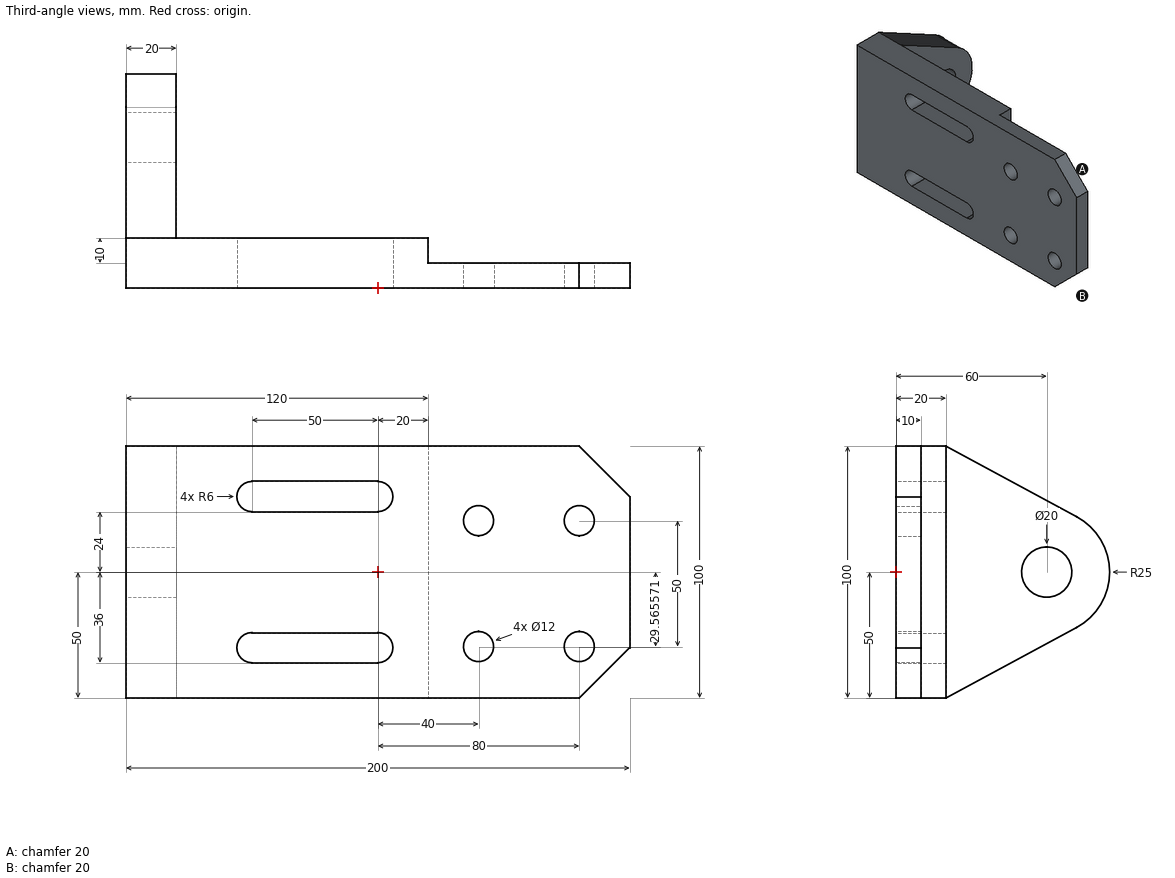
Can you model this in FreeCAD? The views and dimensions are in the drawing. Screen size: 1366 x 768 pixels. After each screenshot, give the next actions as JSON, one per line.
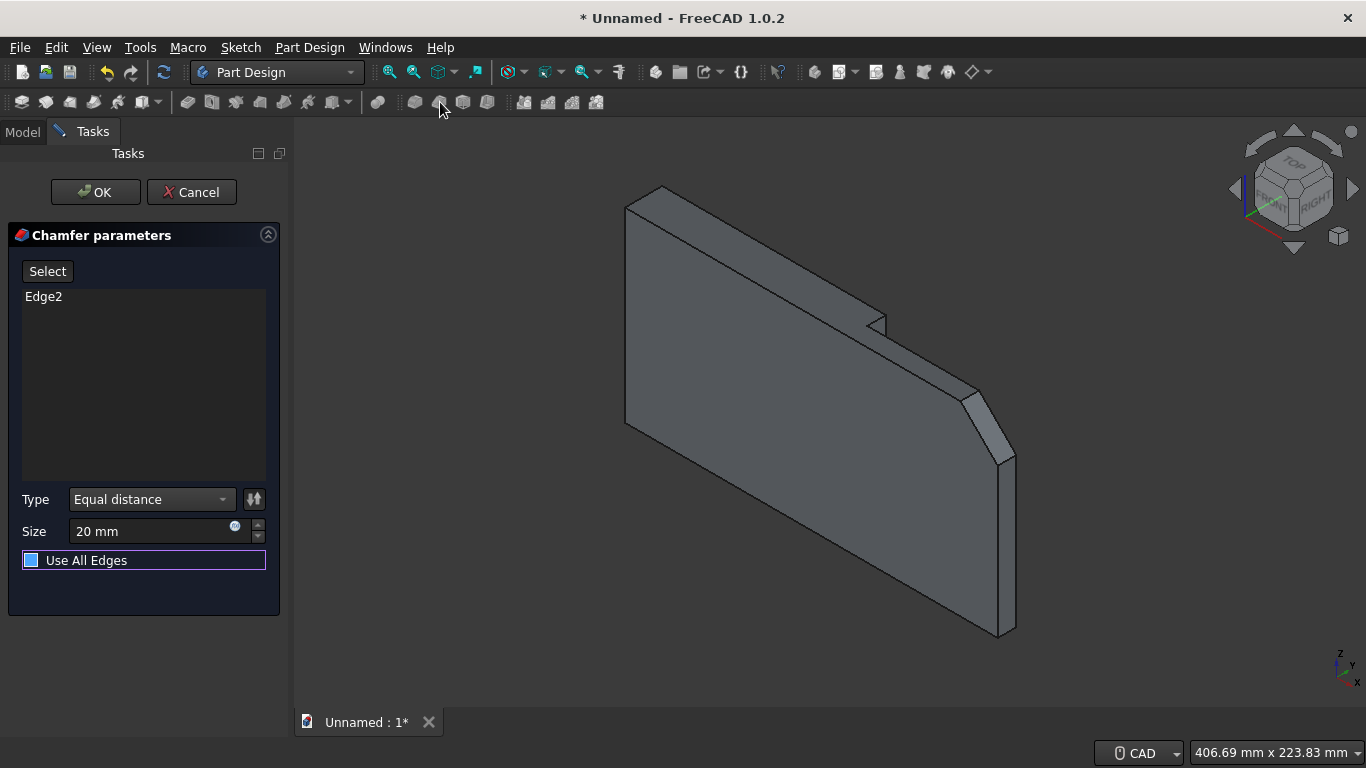
{"action": "left_click", "coordinate": [96, 192]}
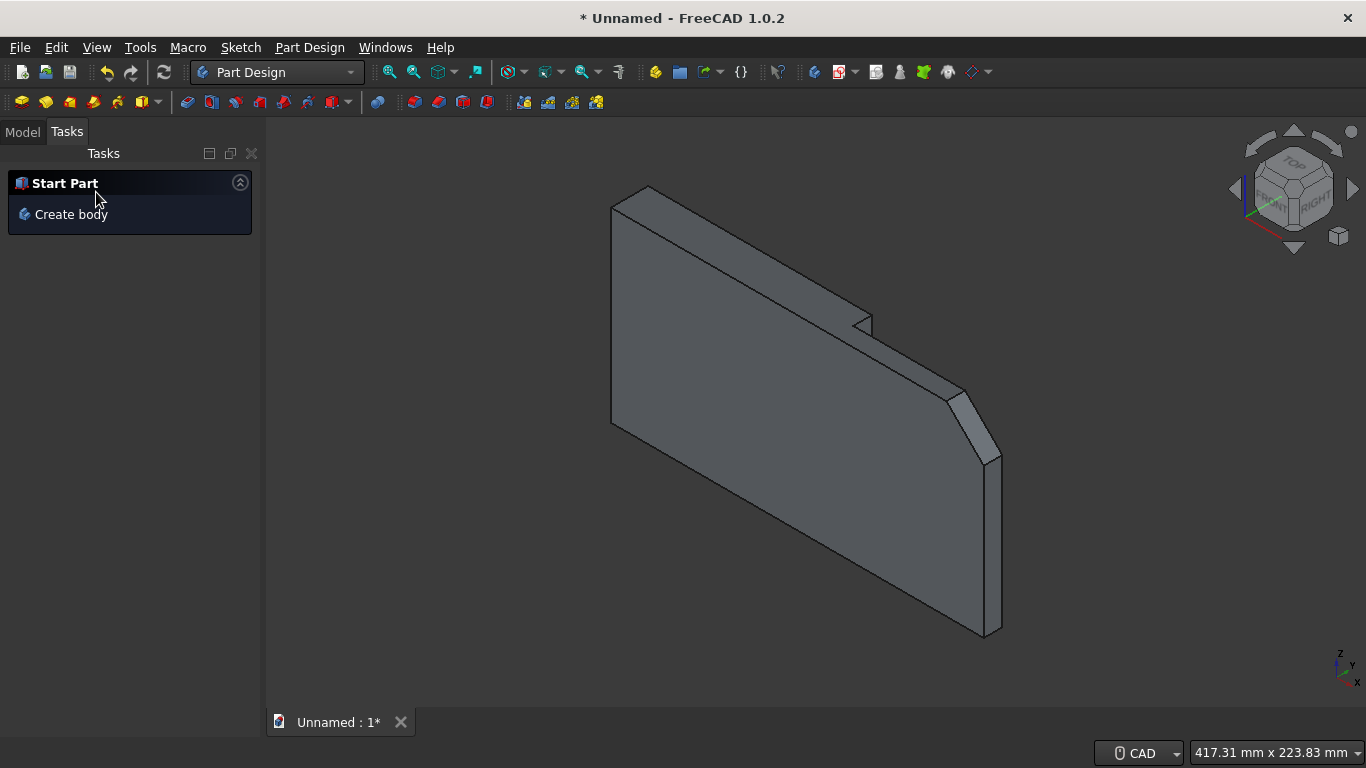
{"action": "key", "text": "2"}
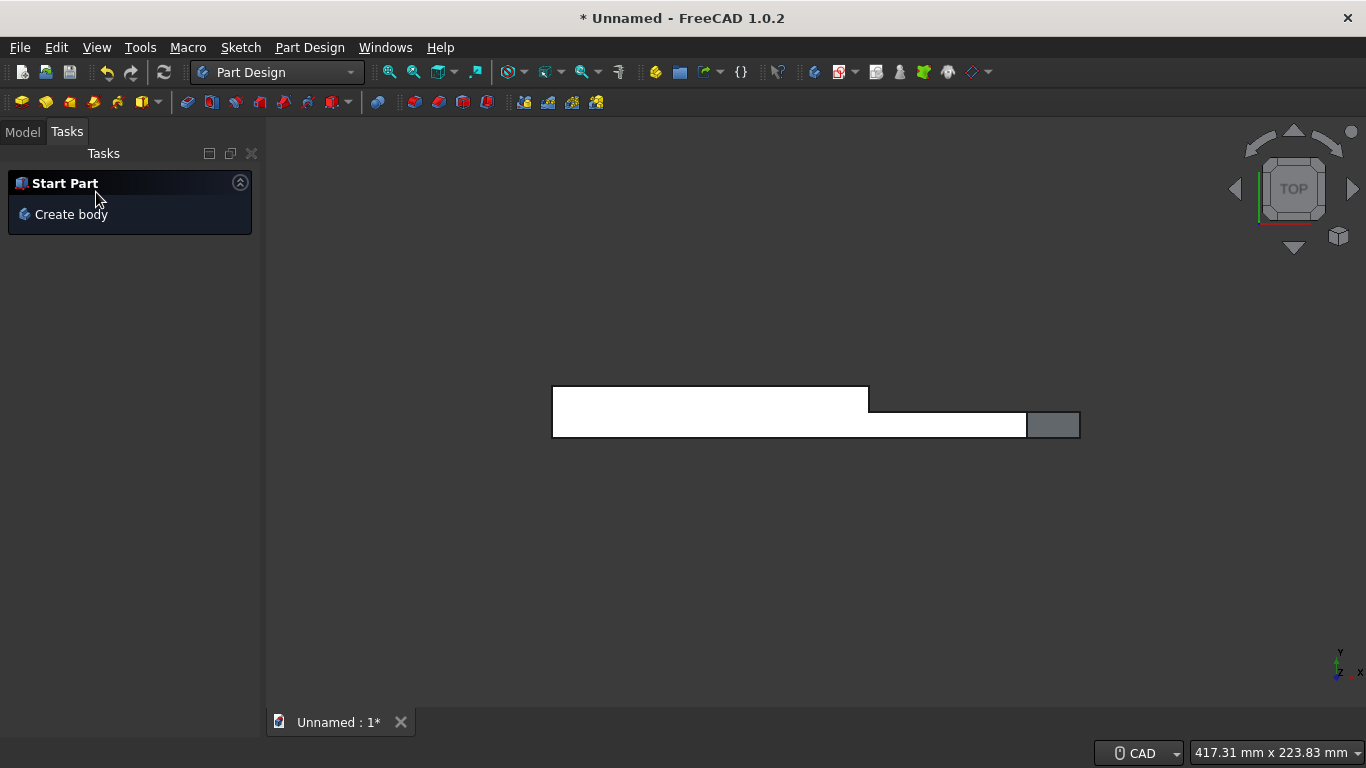
{"action": "key", "text": "0"}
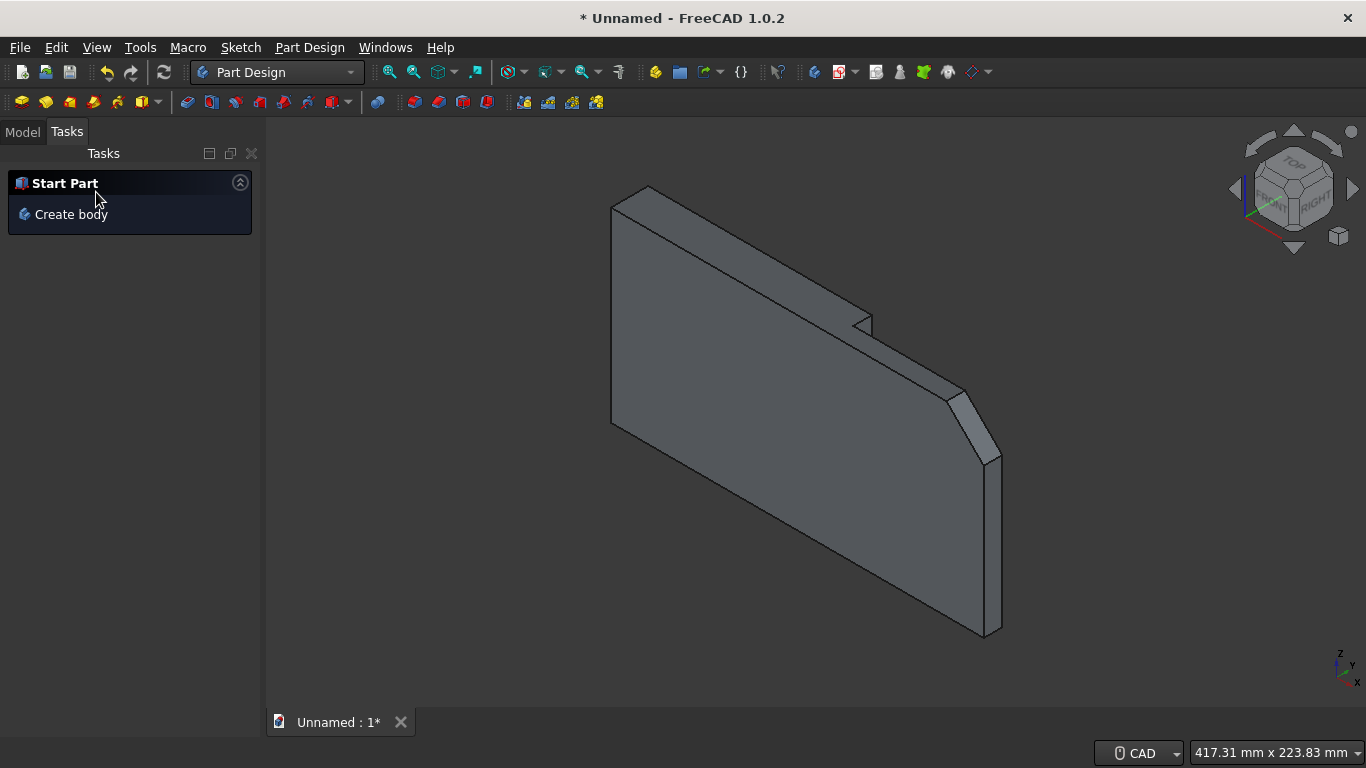
{"action": "key", "text": "1"}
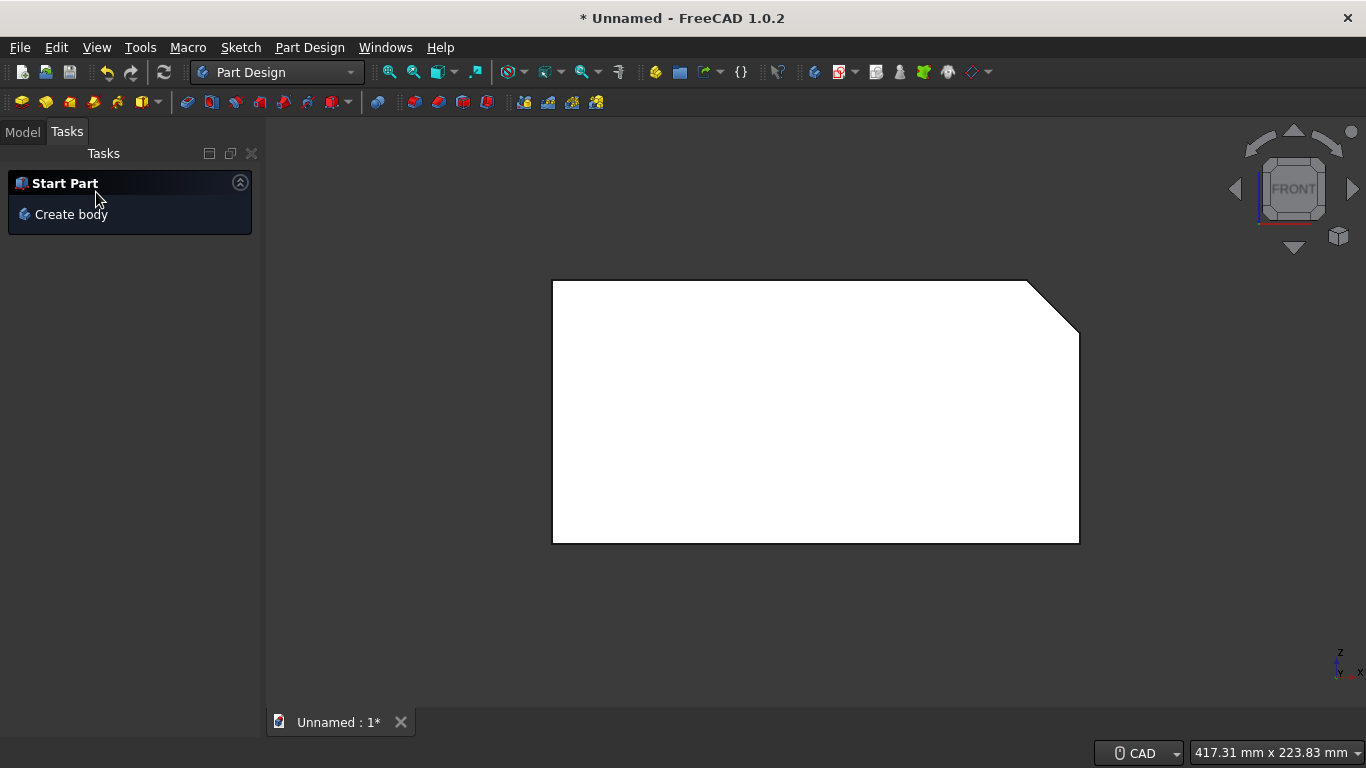
{"action": "key", "text": "3"}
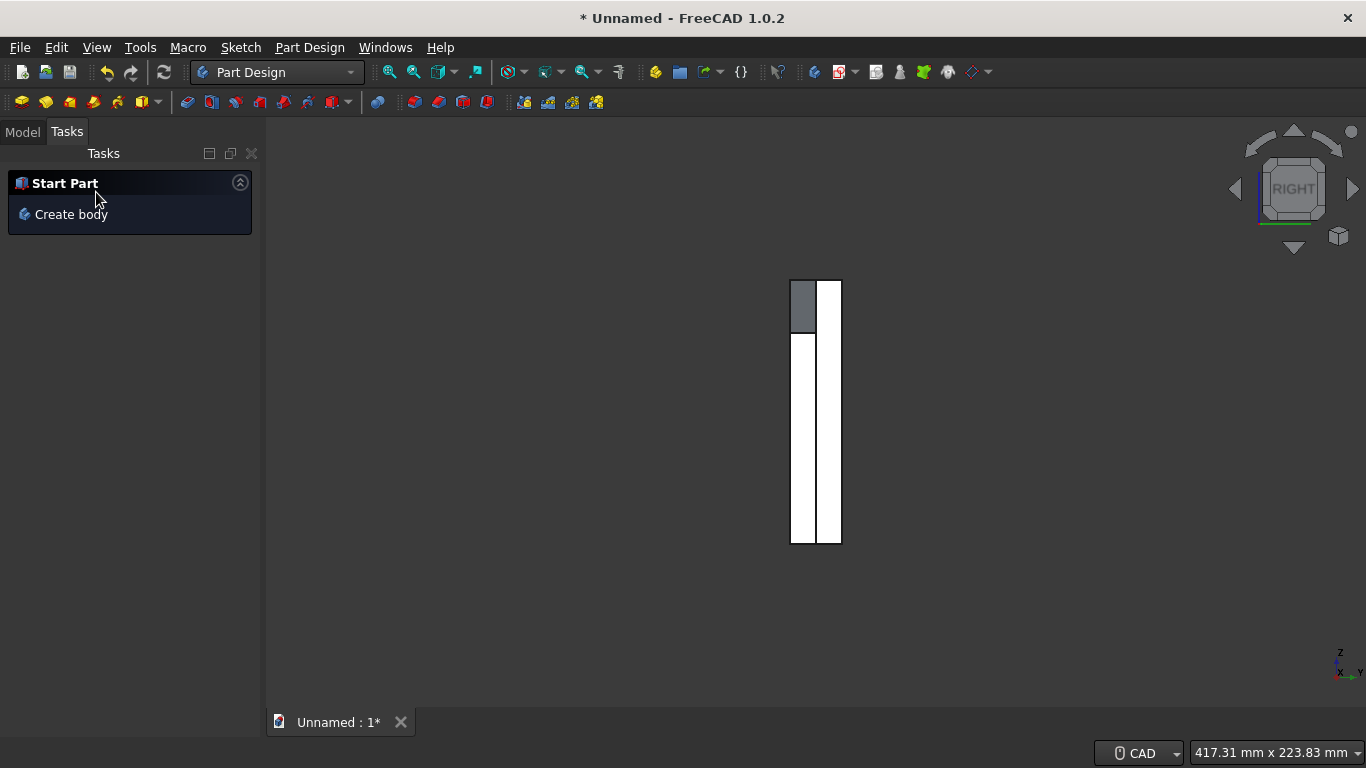
{"action": "left_click", "coordinate": [390, 72]}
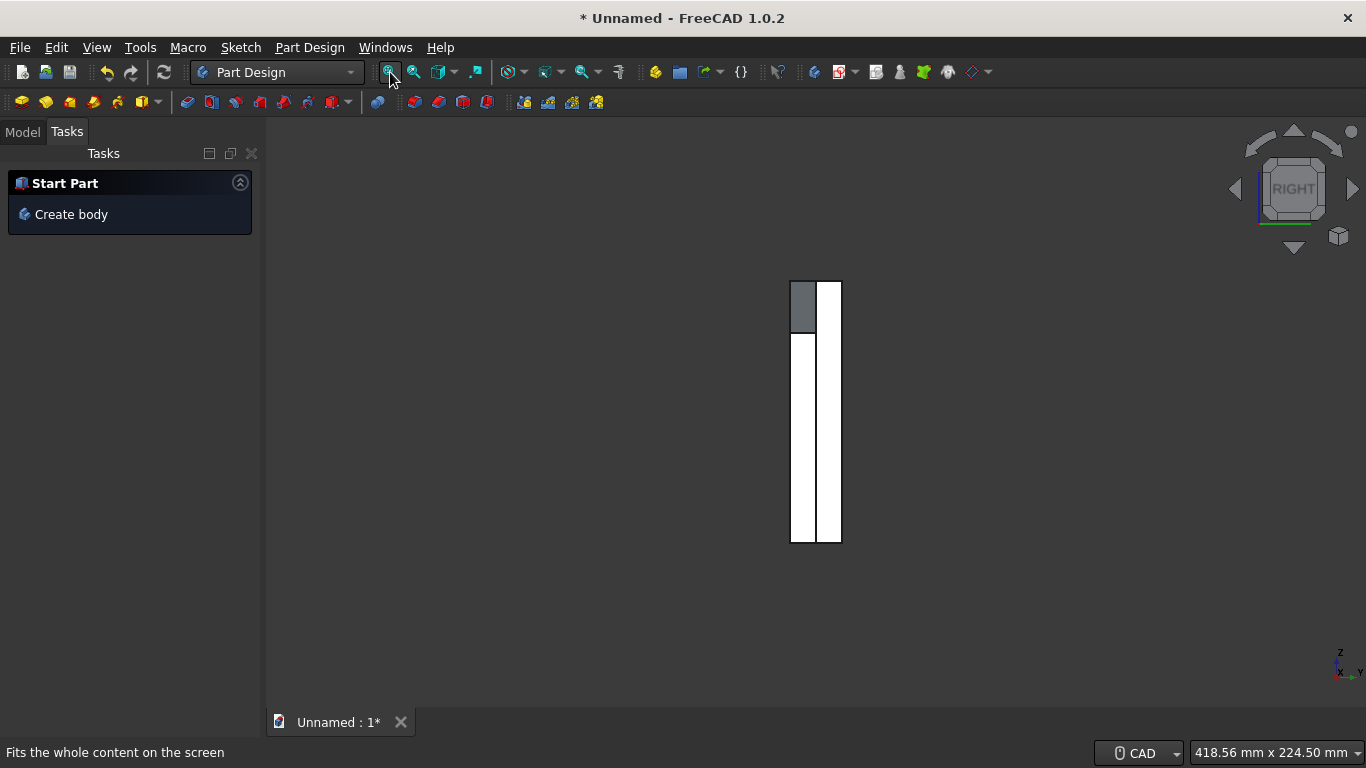
{"action": "left_click", "coordinate": [803, 542]}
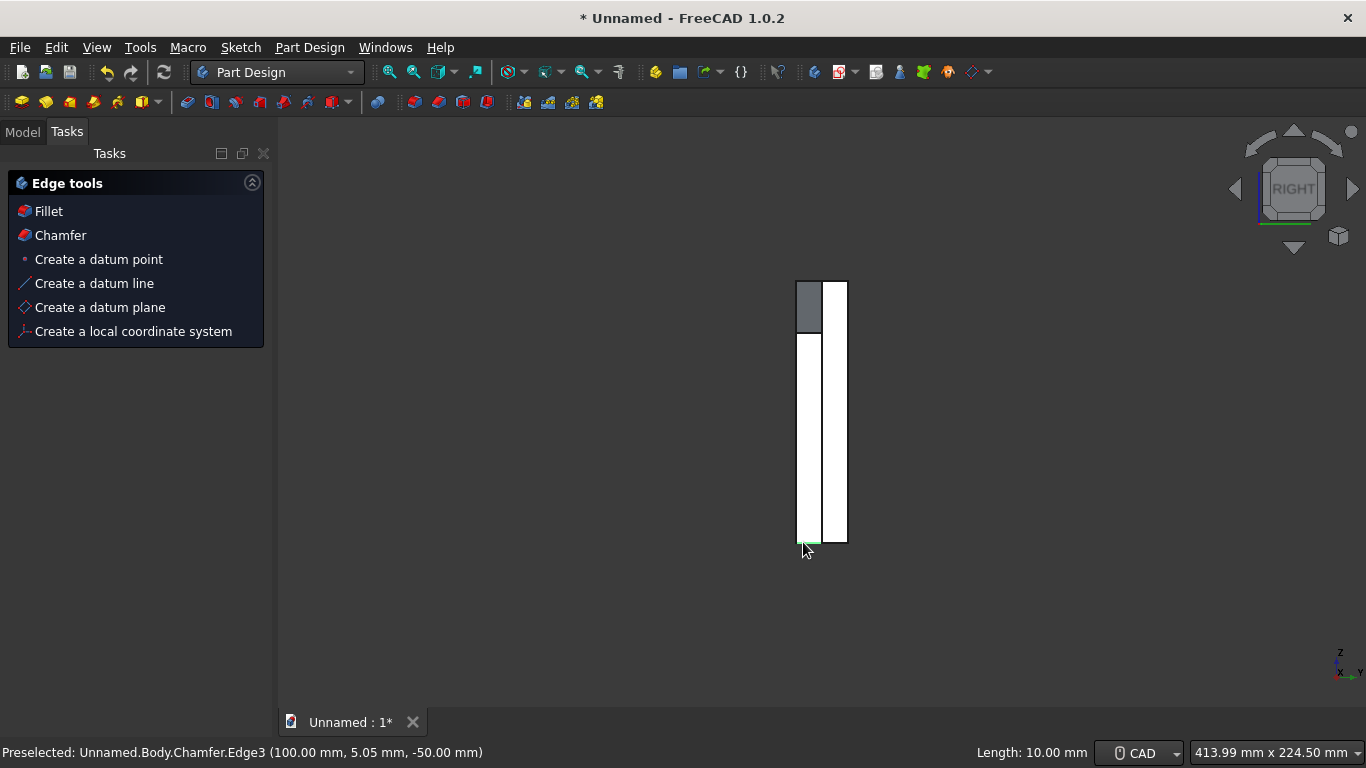
{"action": "left_click", "coordinate": [440, 102]}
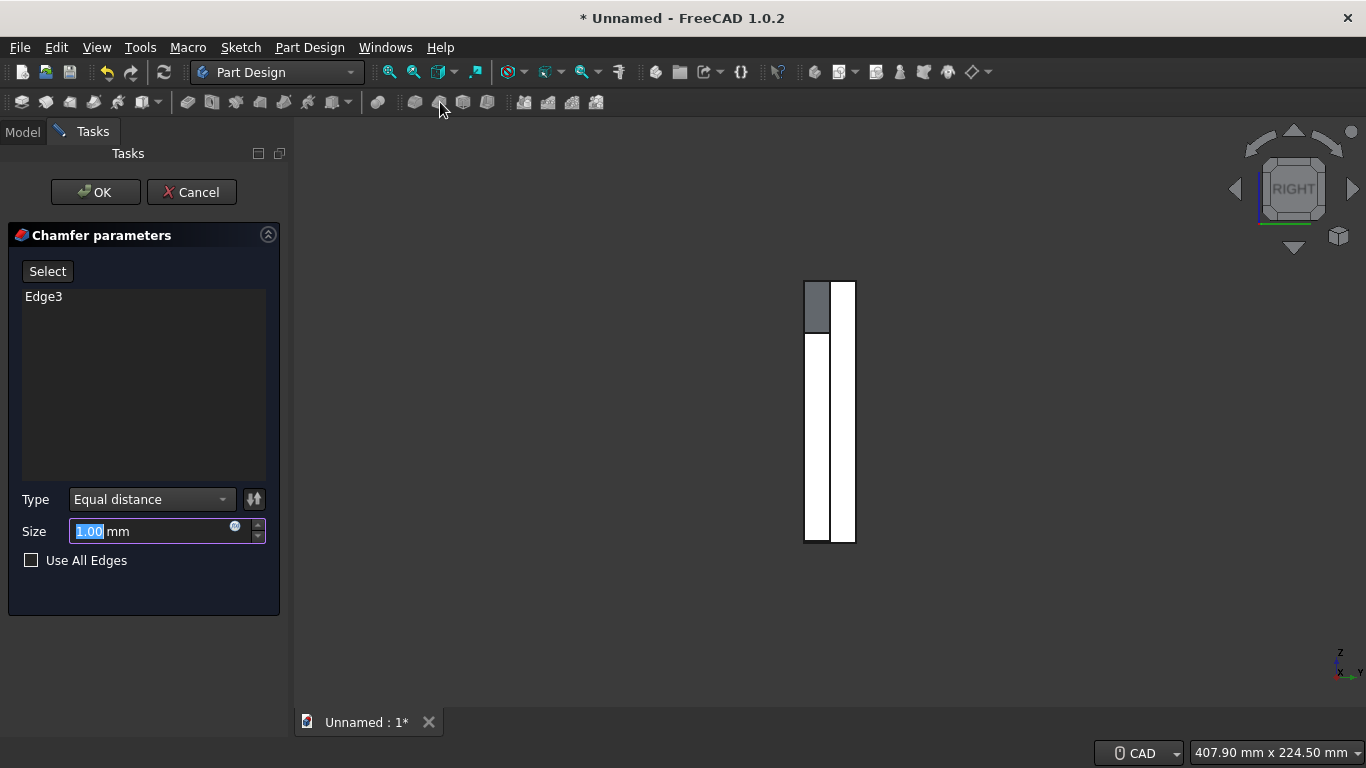
{"action": "type", "text": "20"}
{"action": "key", "text": "Tab"}